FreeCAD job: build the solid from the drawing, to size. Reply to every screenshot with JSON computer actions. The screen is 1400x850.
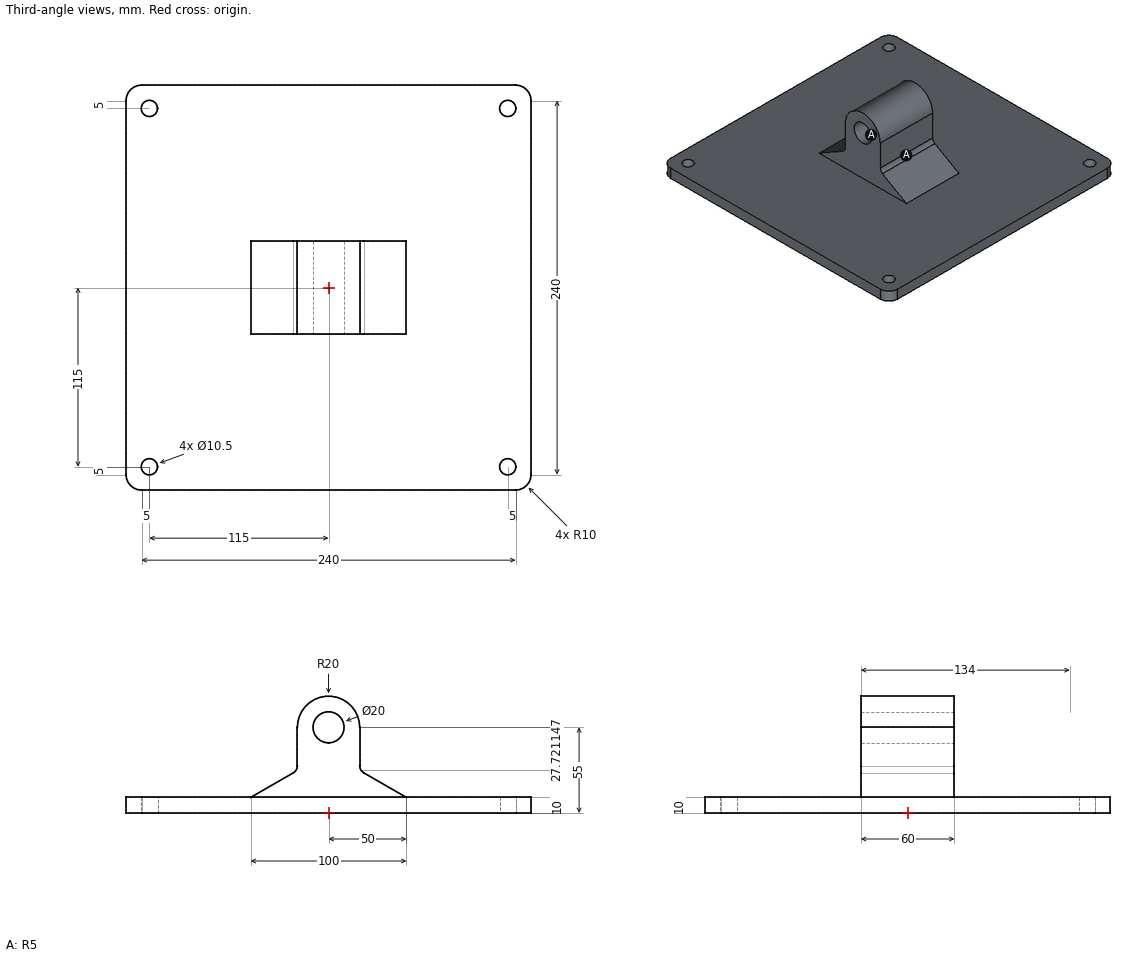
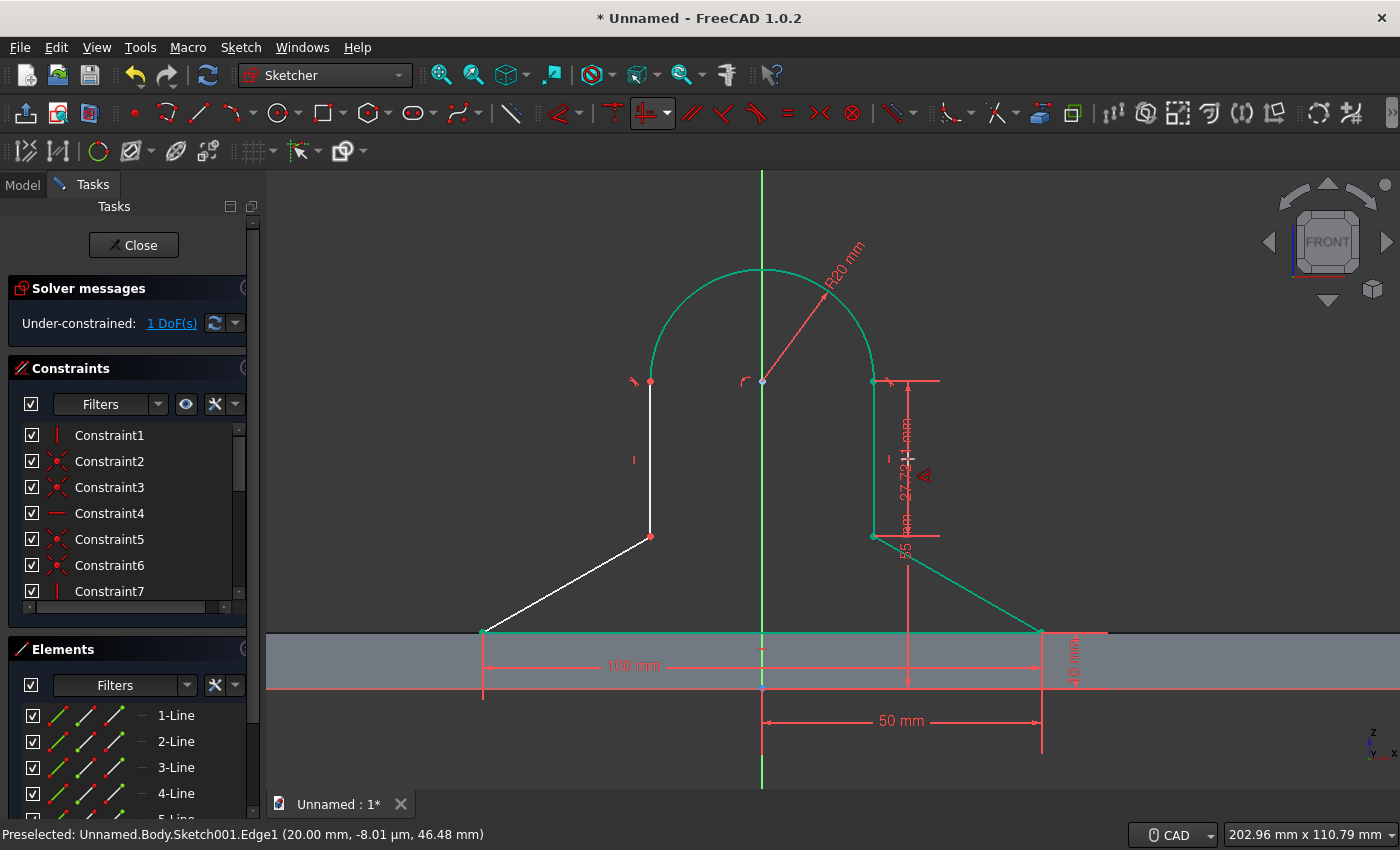
{"action": "left_click", "coordinate": [650, 490]}
{"action": "left_click", "coordinate": [616, 459]}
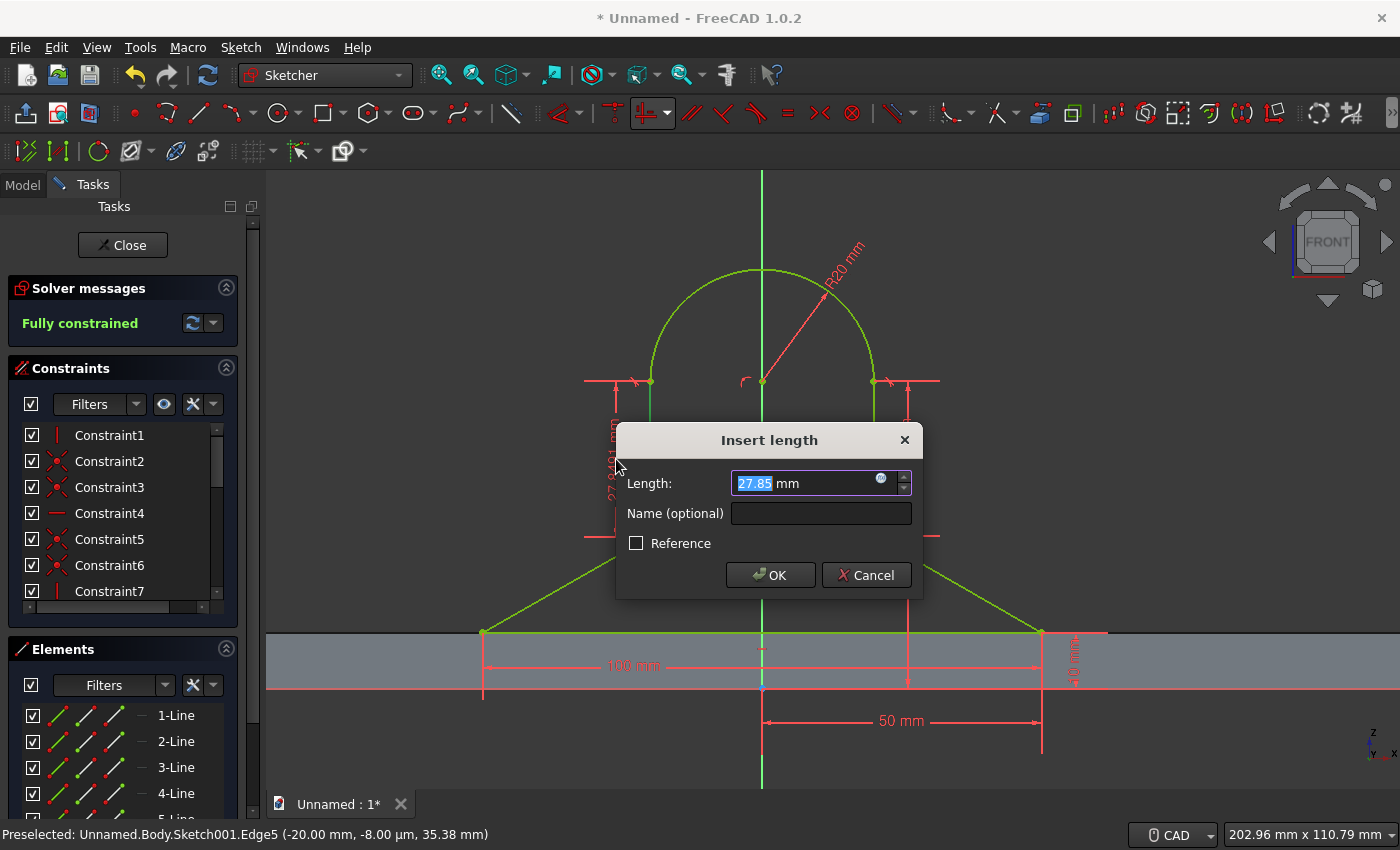
{"action": "type", "text": "27.721147"}
{"action": "key", "text": "Return"}
{"action": "key", "text": "Escape"}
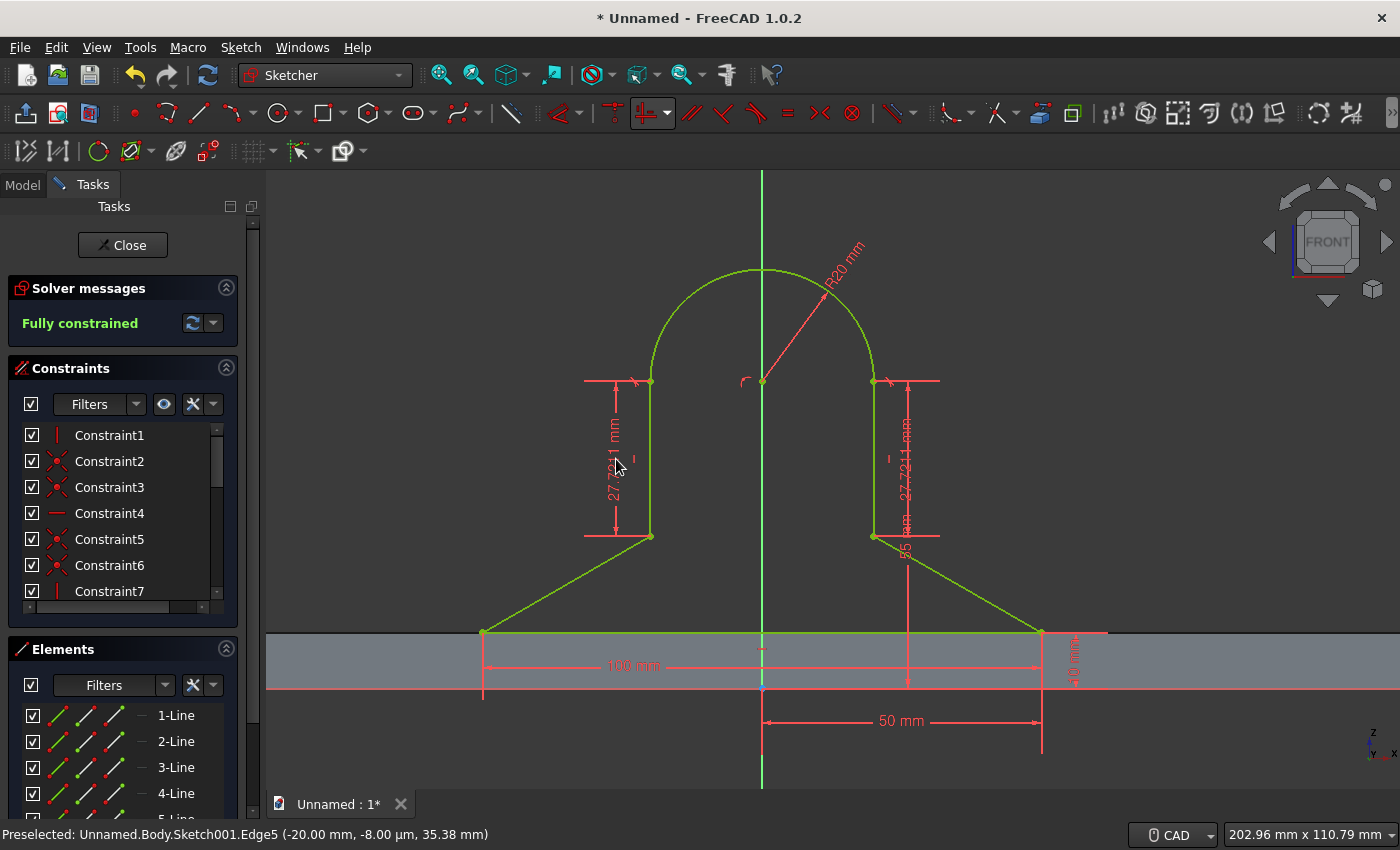
{"action": "left_click", "coordinate": [123, 245]}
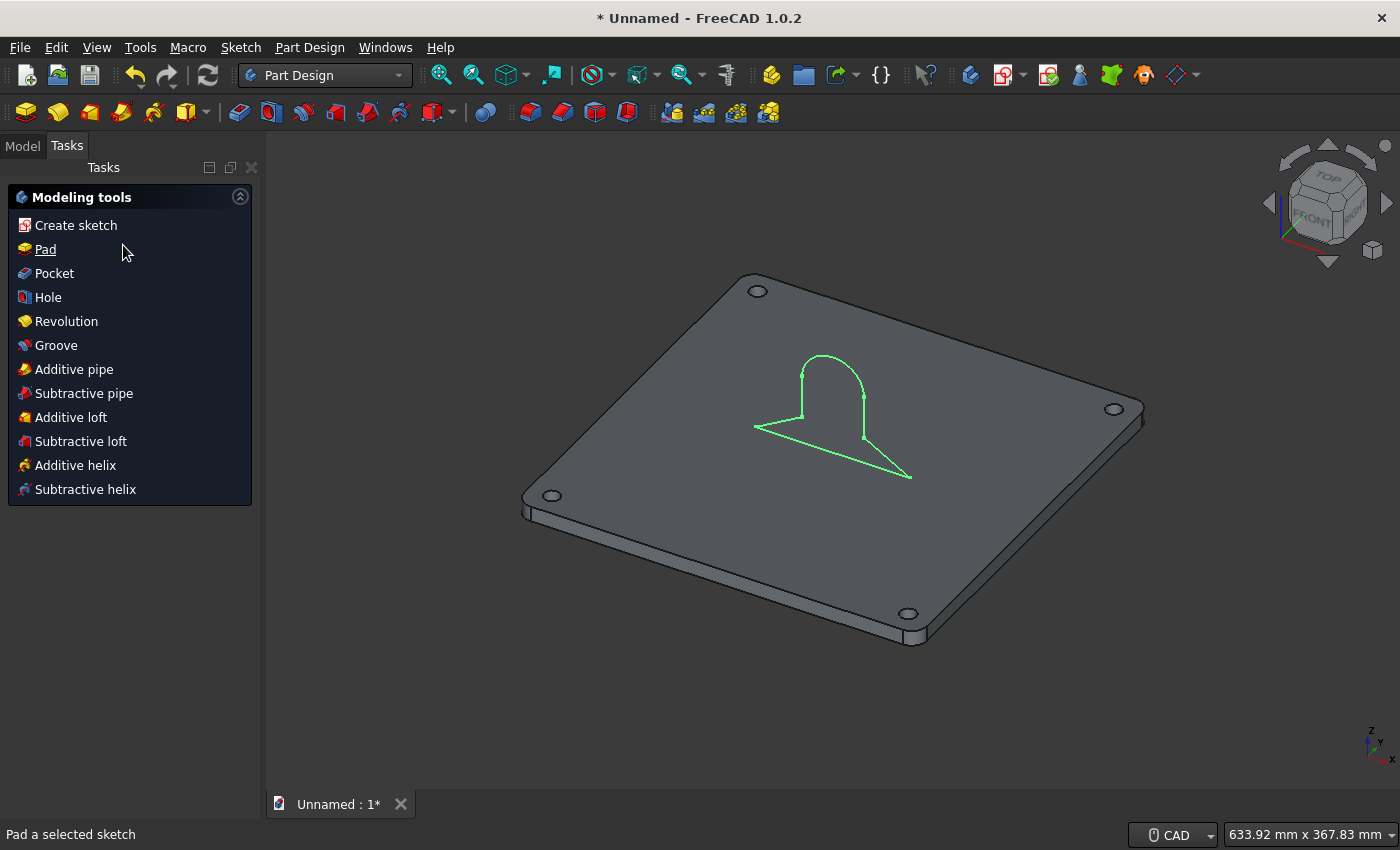
{"action": "left_click", "coordinate": [26, 112]}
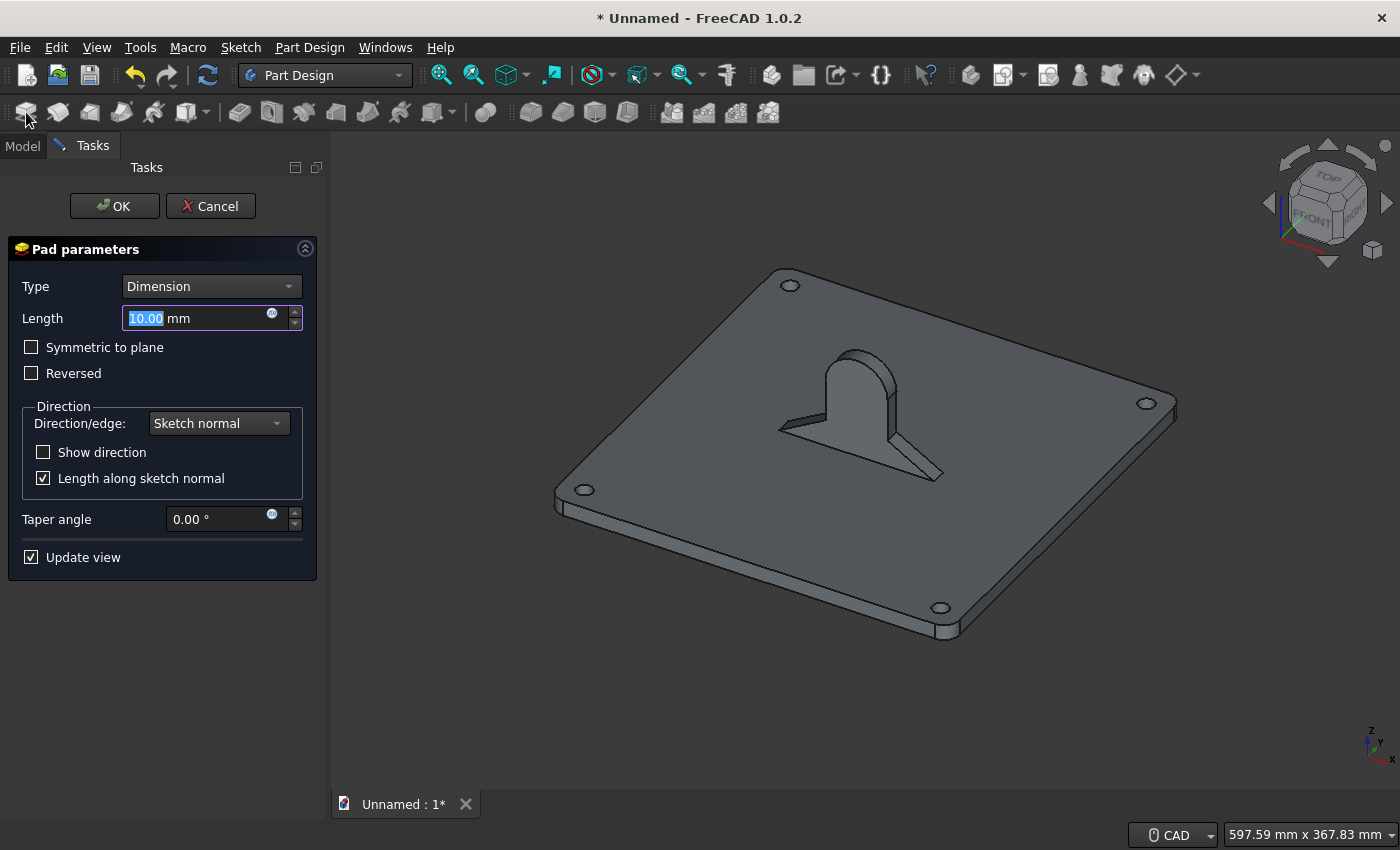
{"action": "type", "text": "60"}
{"action": "key", "text": "Tab"}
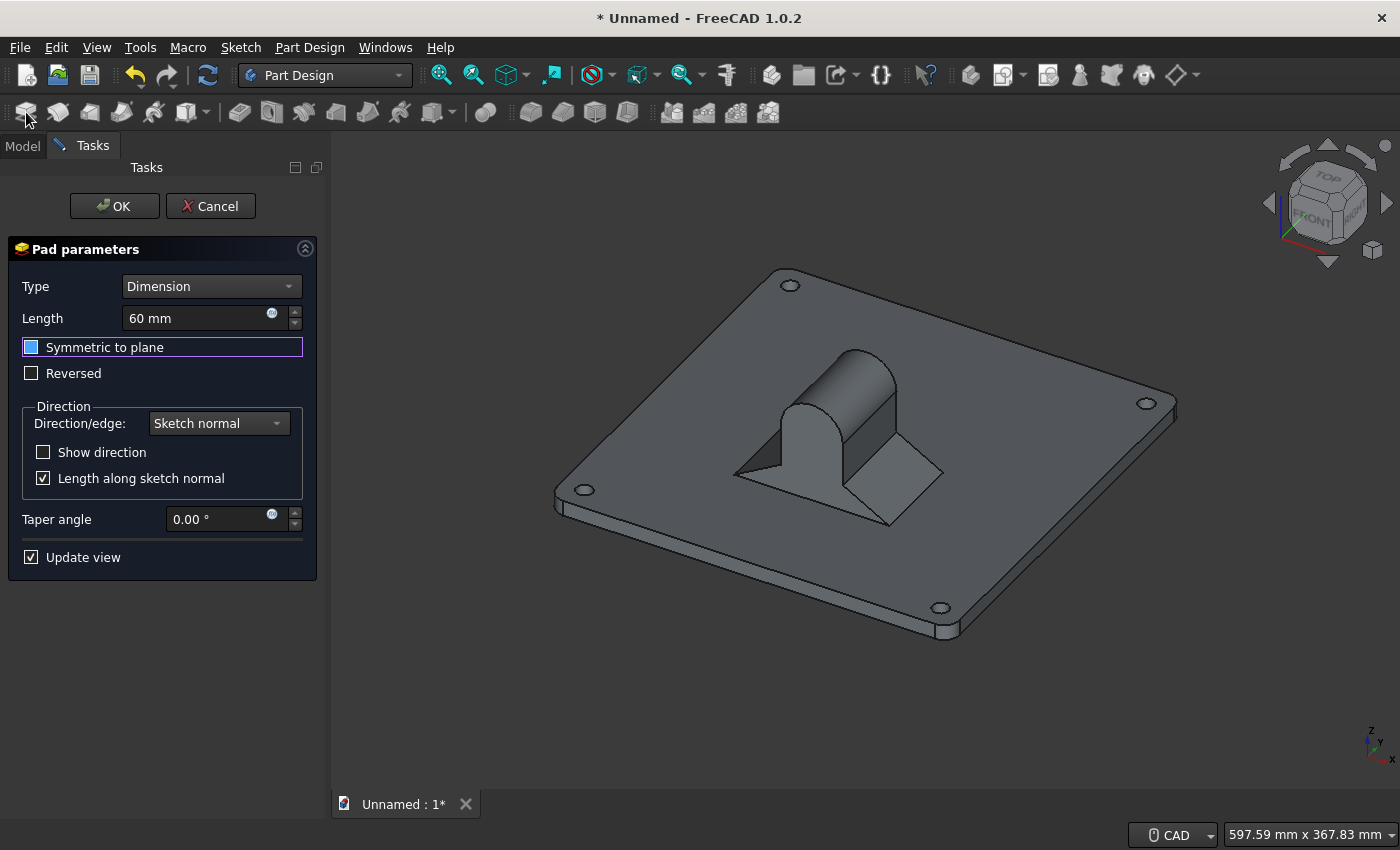
{"action": "left_click", "coordinate": [30, 347]}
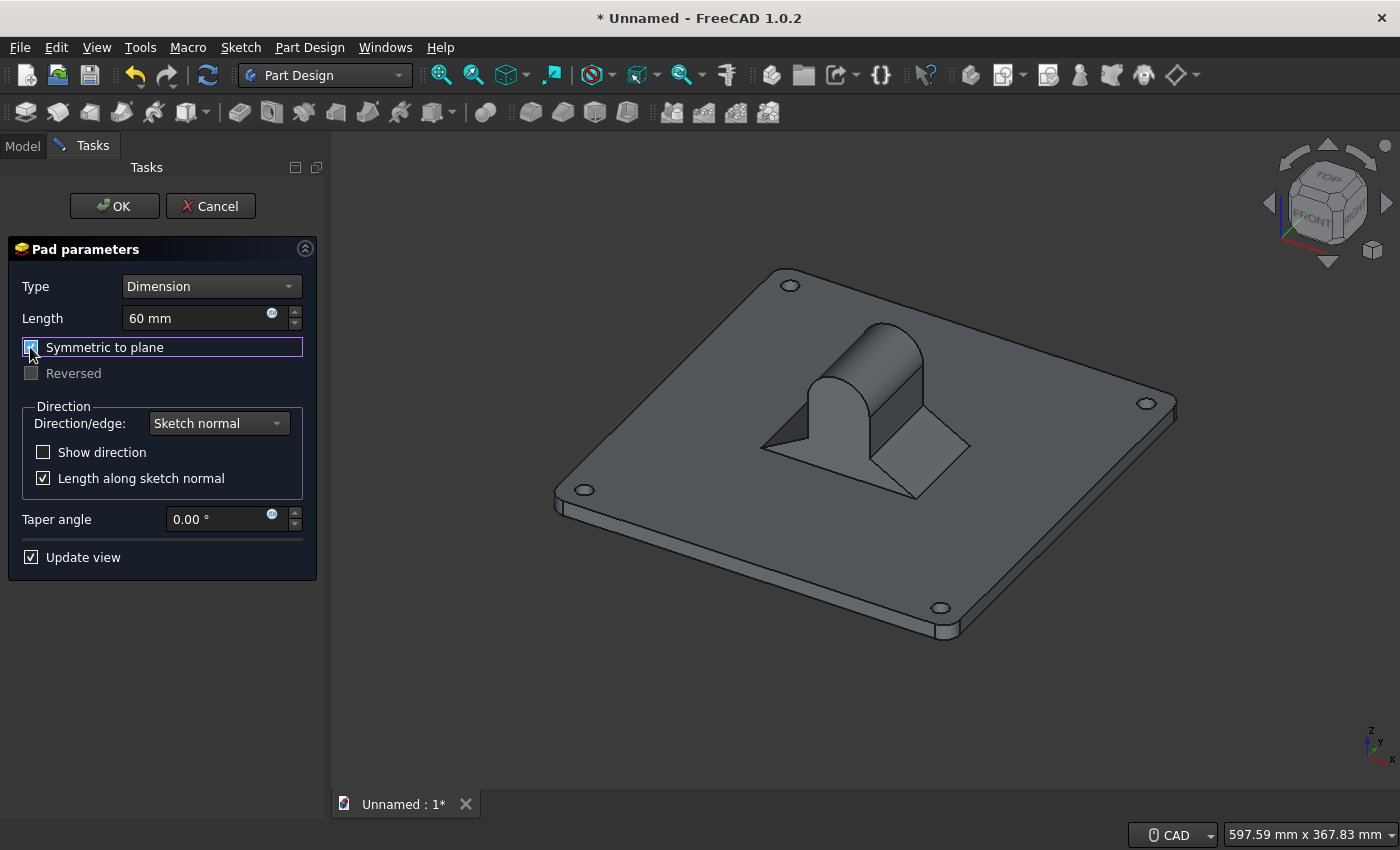
{"action": "left_click", "coordinate": [115, 206]}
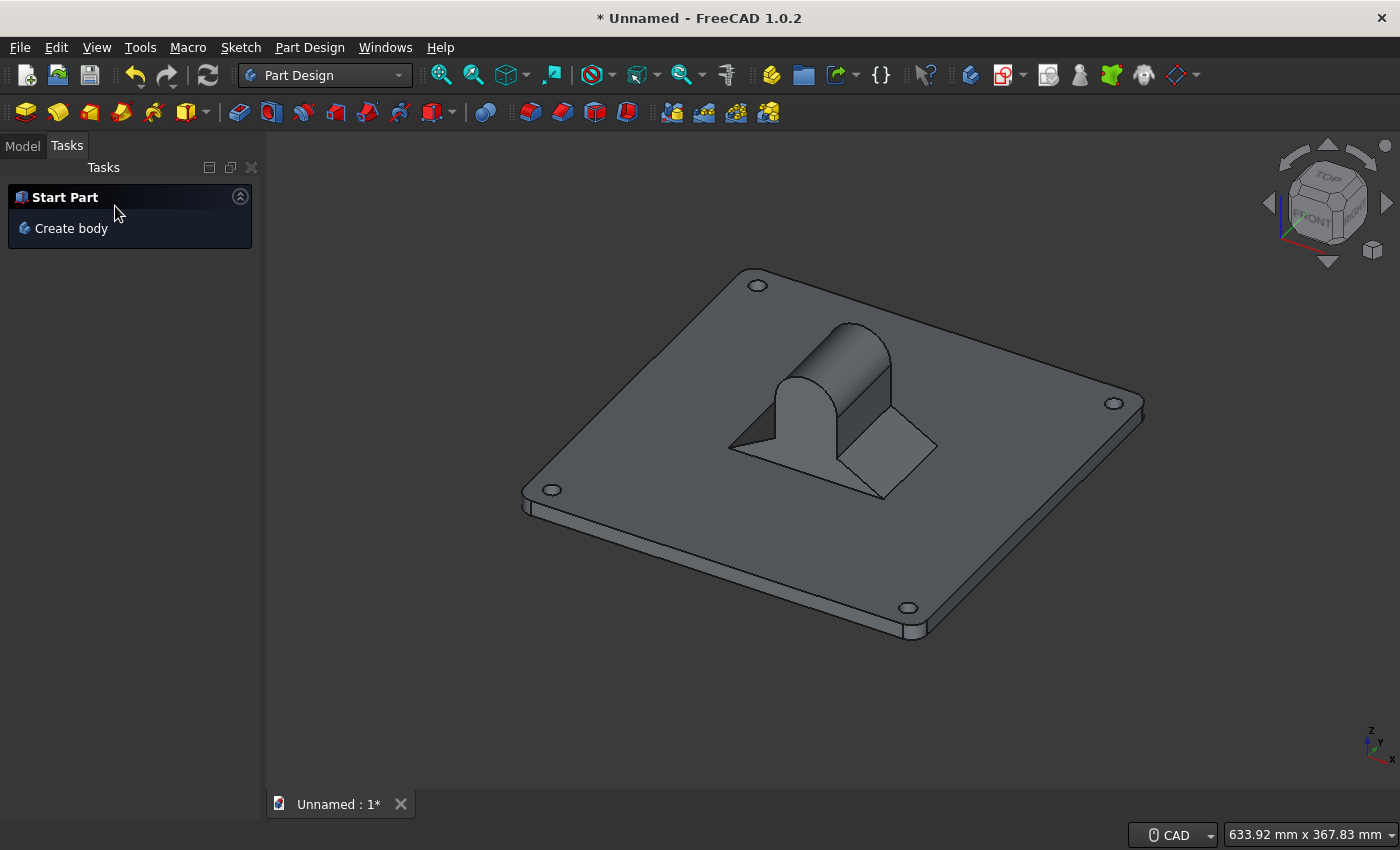
{"action": "left_click", "coordinate": [806, 411]}